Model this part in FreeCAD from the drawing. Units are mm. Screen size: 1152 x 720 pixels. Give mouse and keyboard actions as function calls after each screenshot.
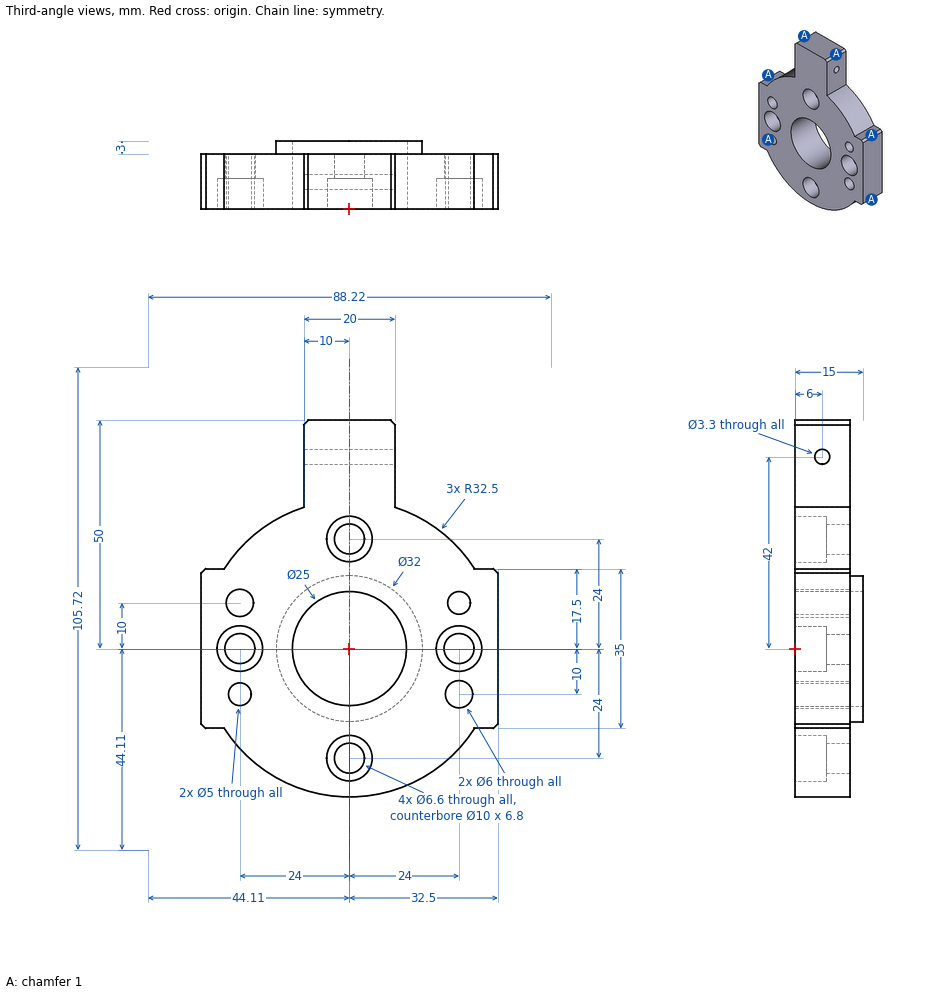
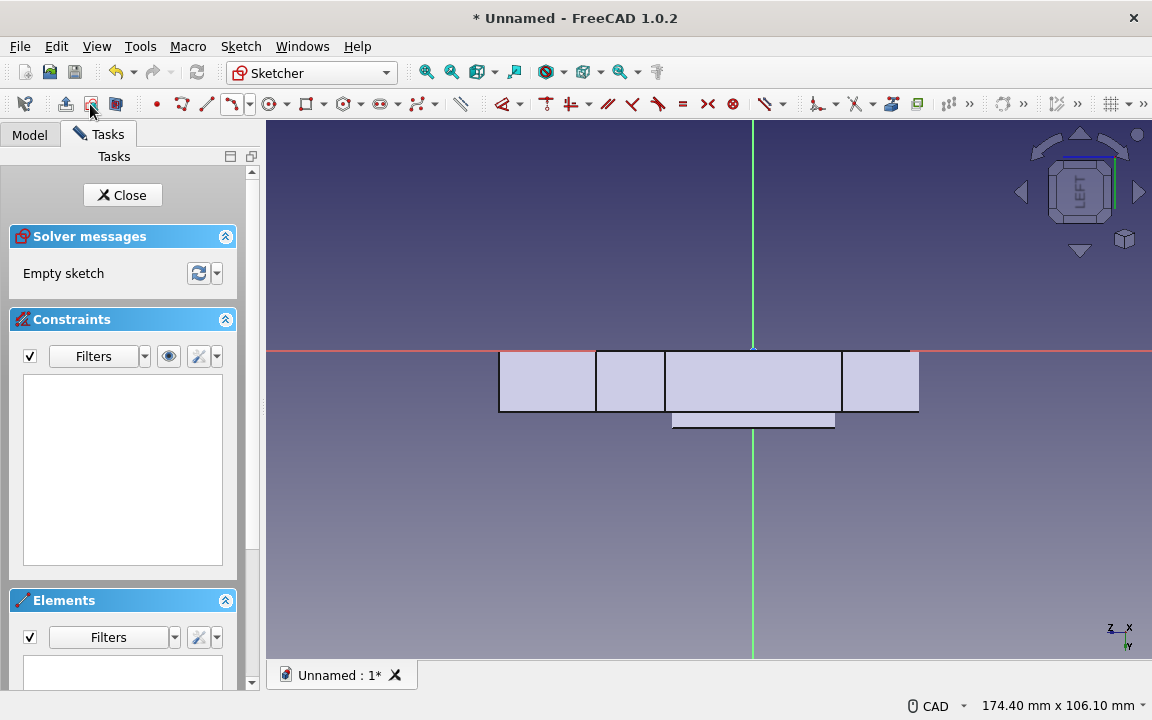
click(116, 104)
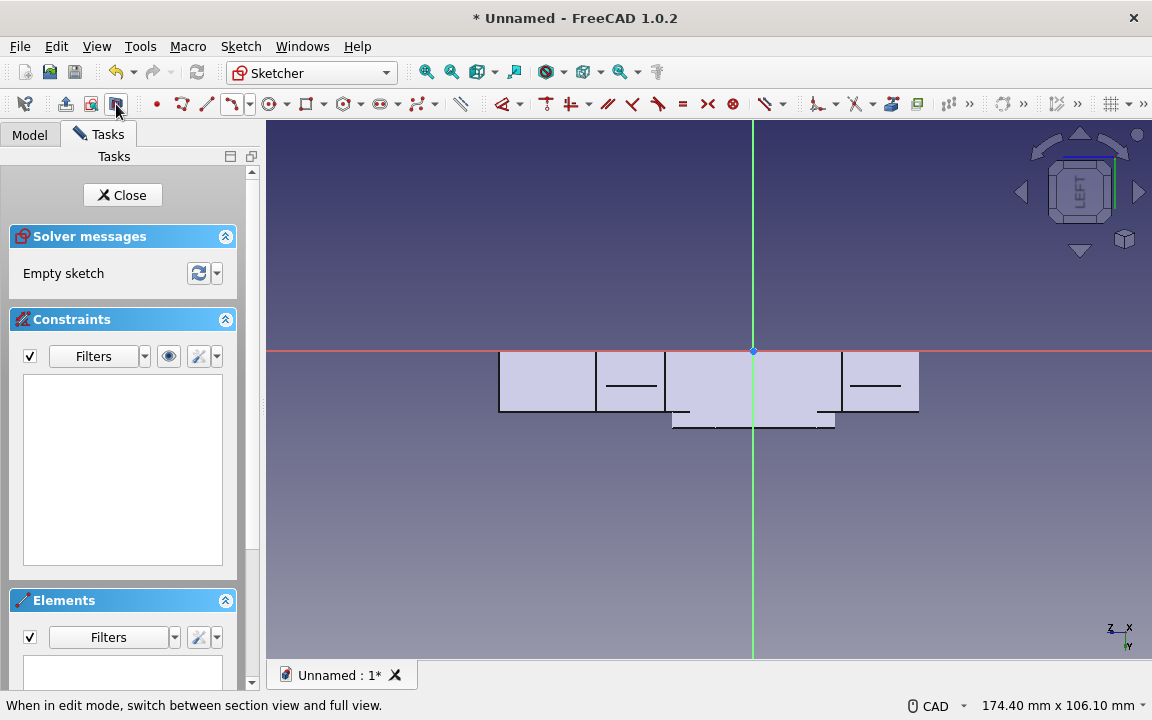
scroll(535, 381, up, 15)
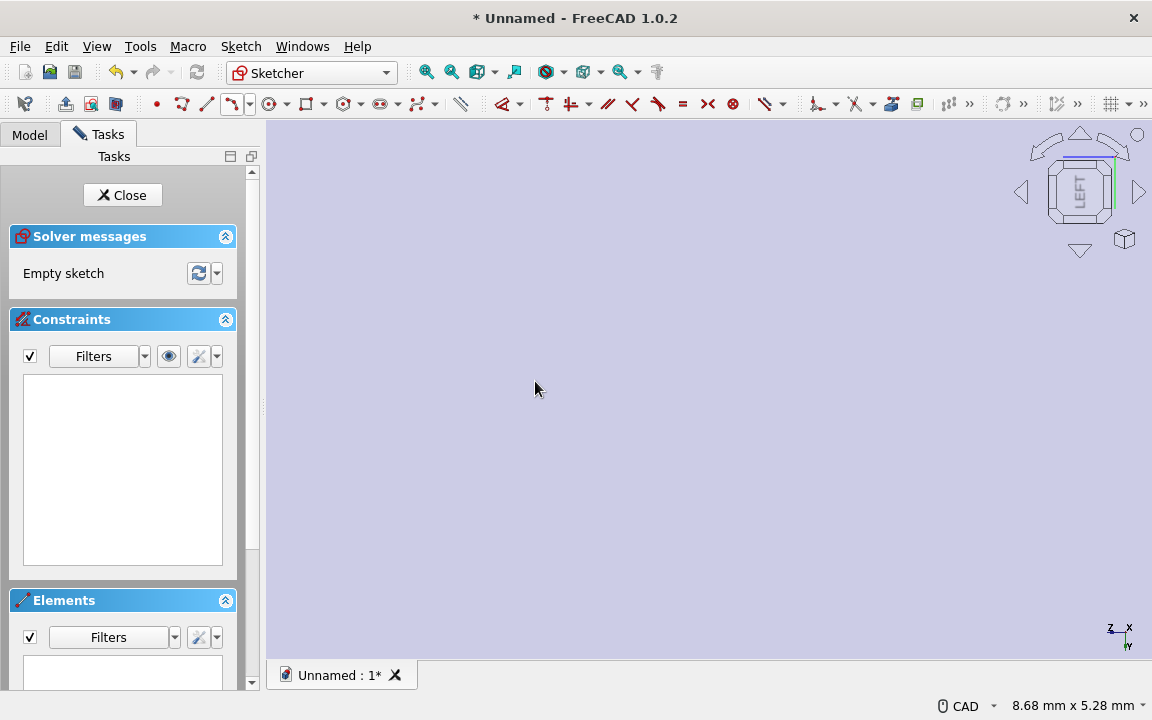
click(268, 104)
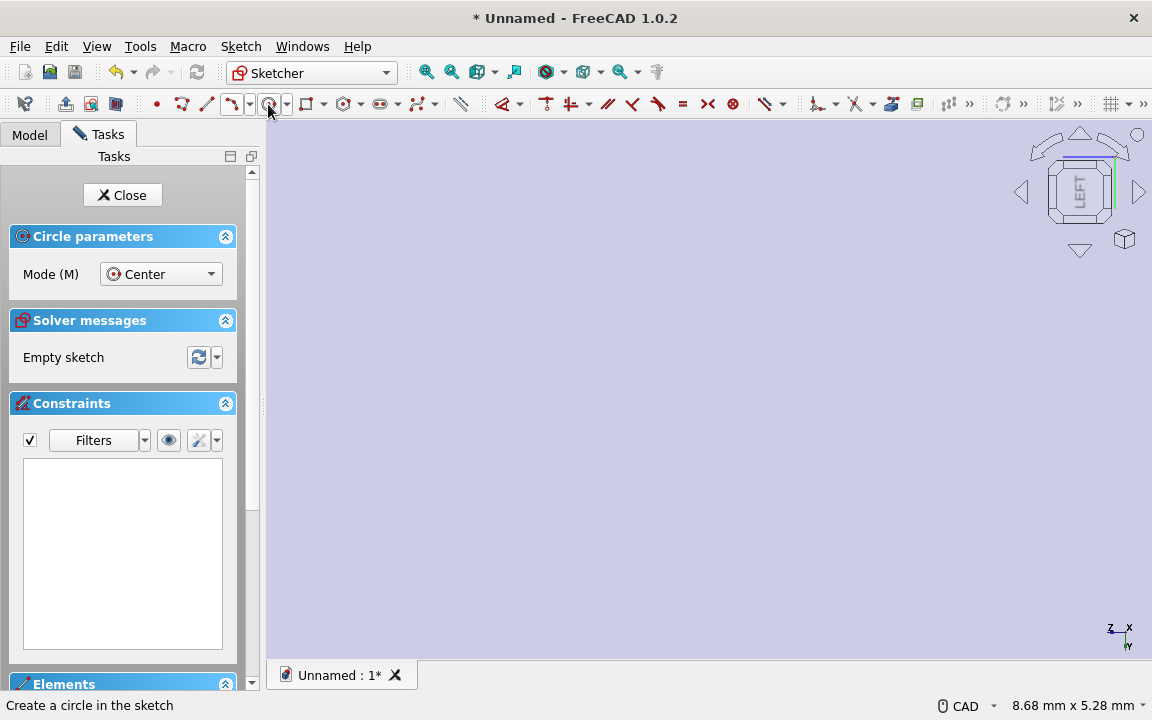
click(631, 389)
click(750, 270)
key(Escape)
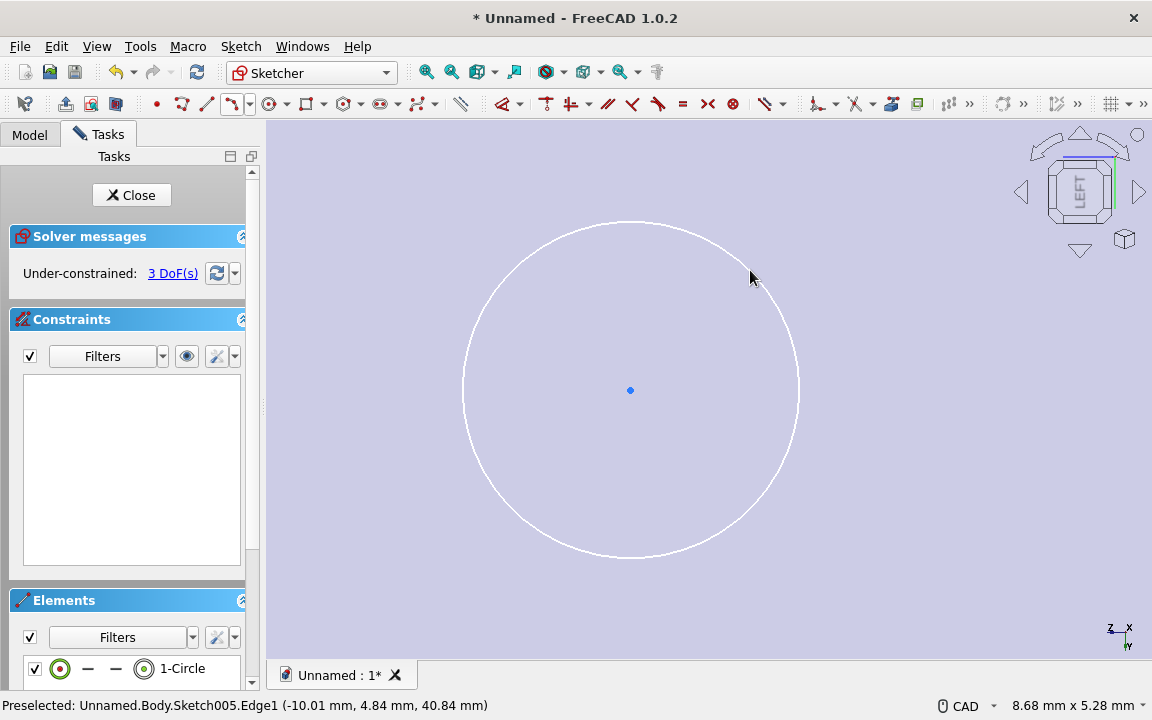
key(d)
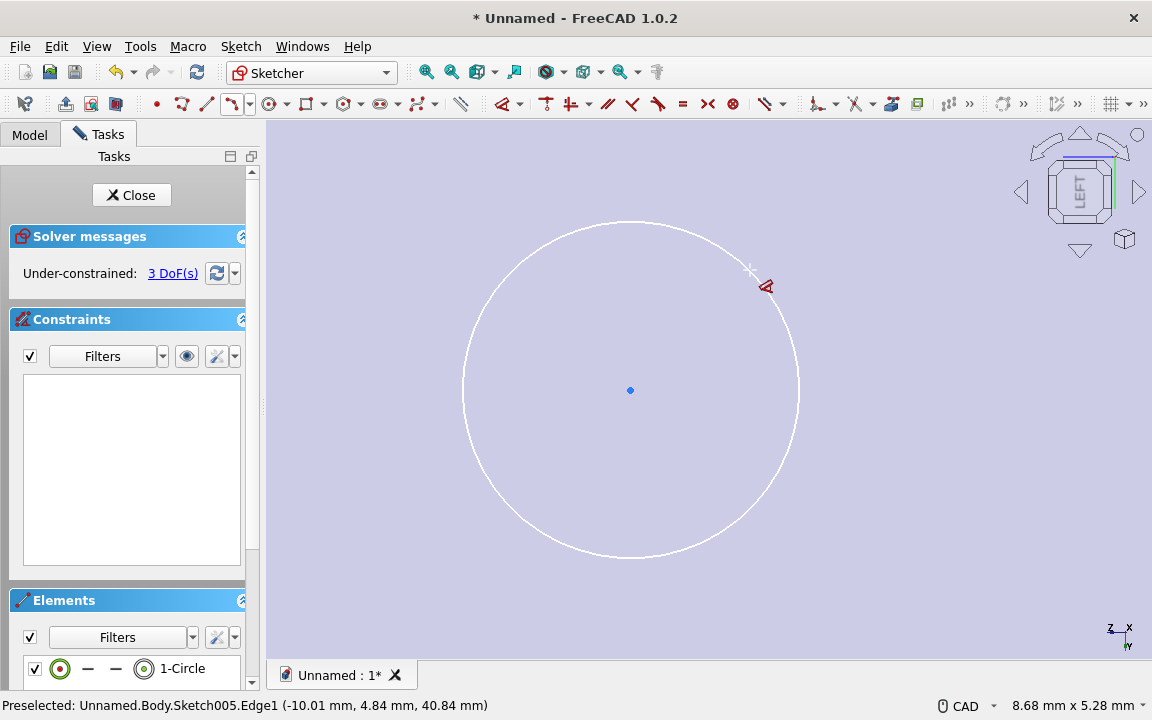
click(750, 271)
click(773, 248)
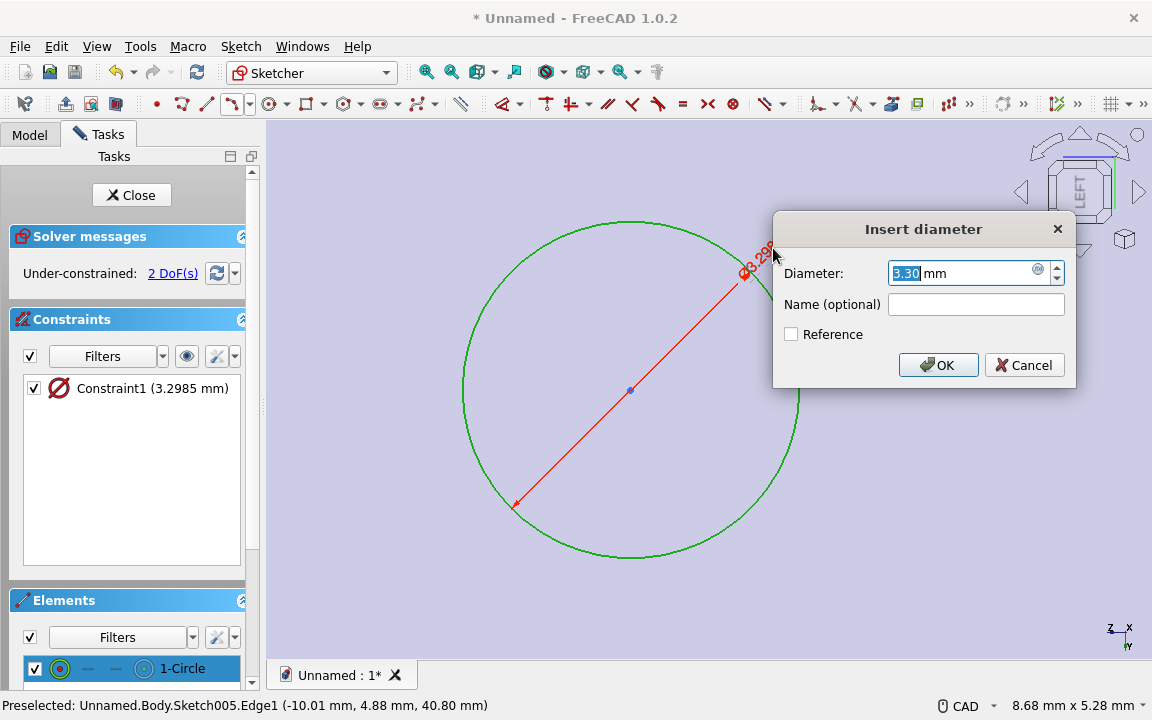
text(3.3)
key(Return)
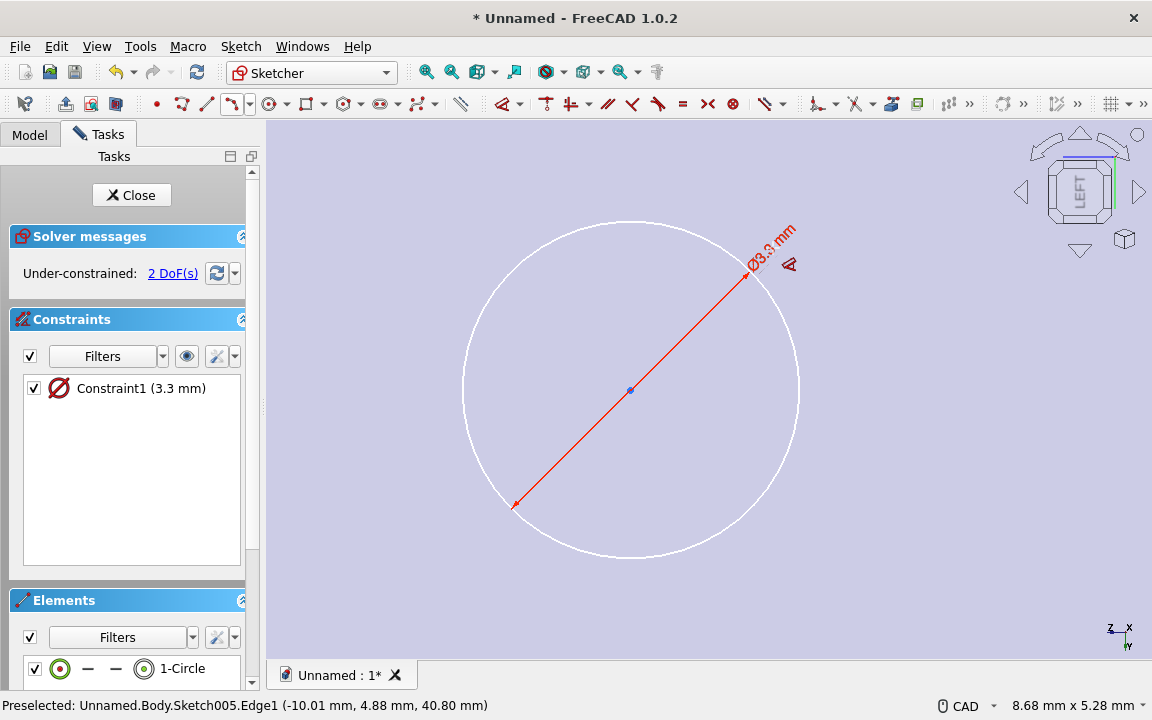
click(631, 390)
click(597, 269)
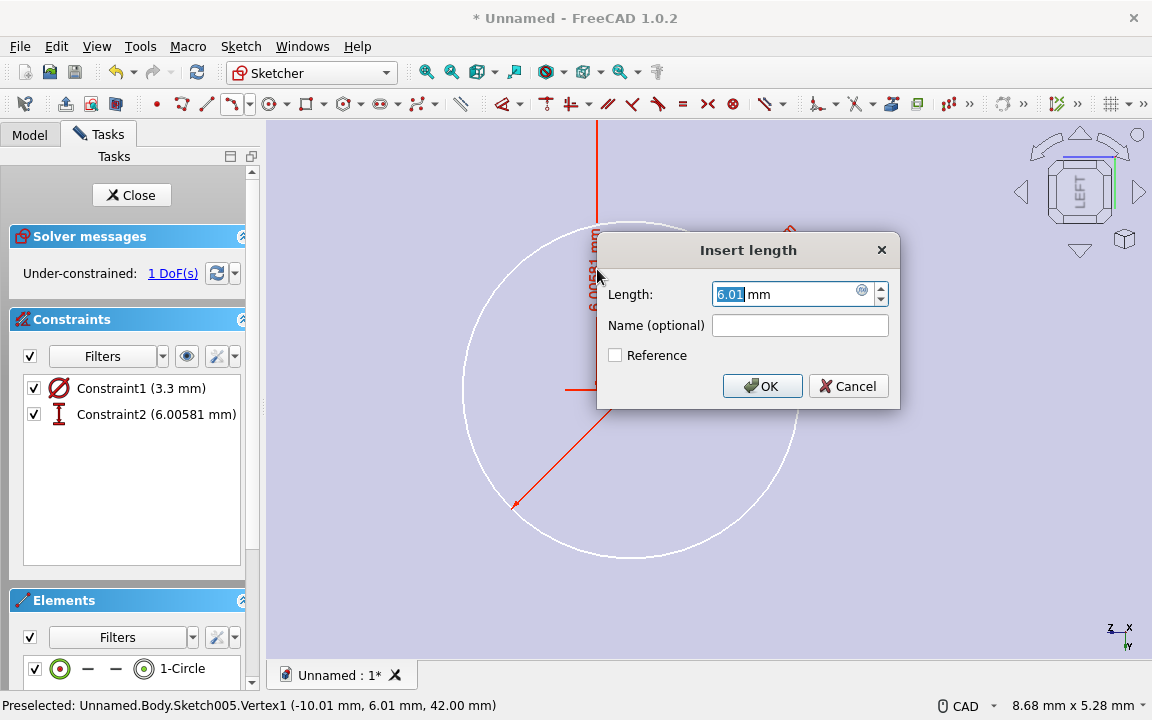
text(6)
key(Return)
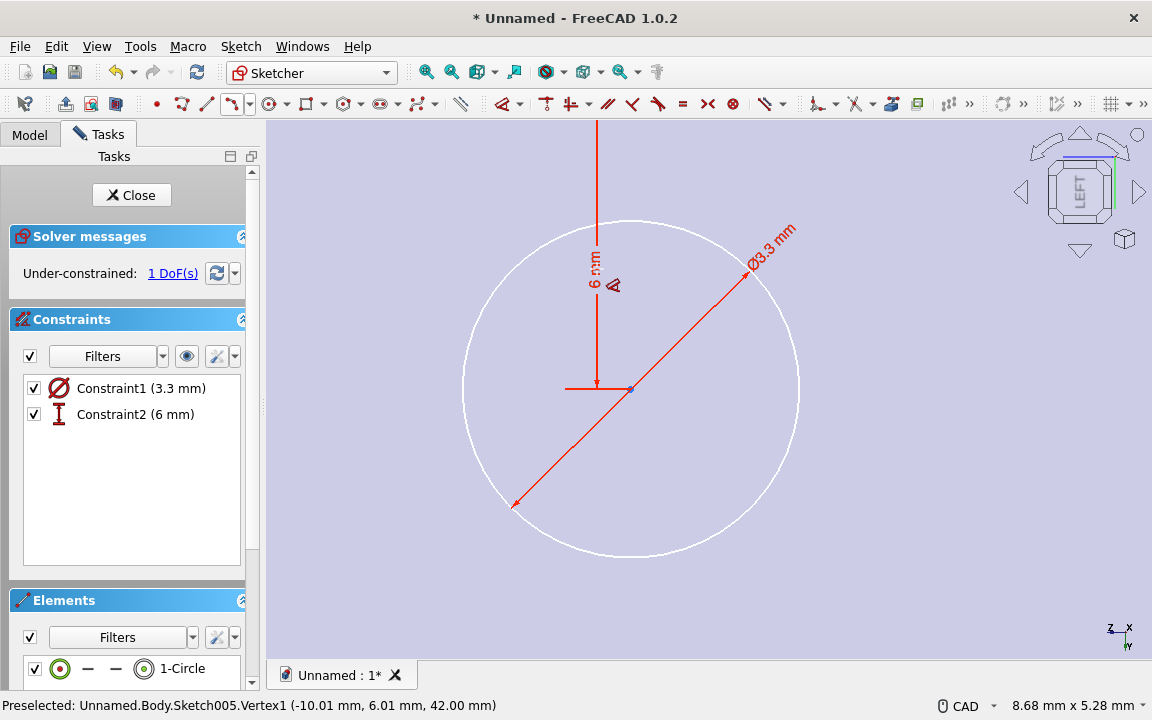
click(631, 389)
click(727, 423)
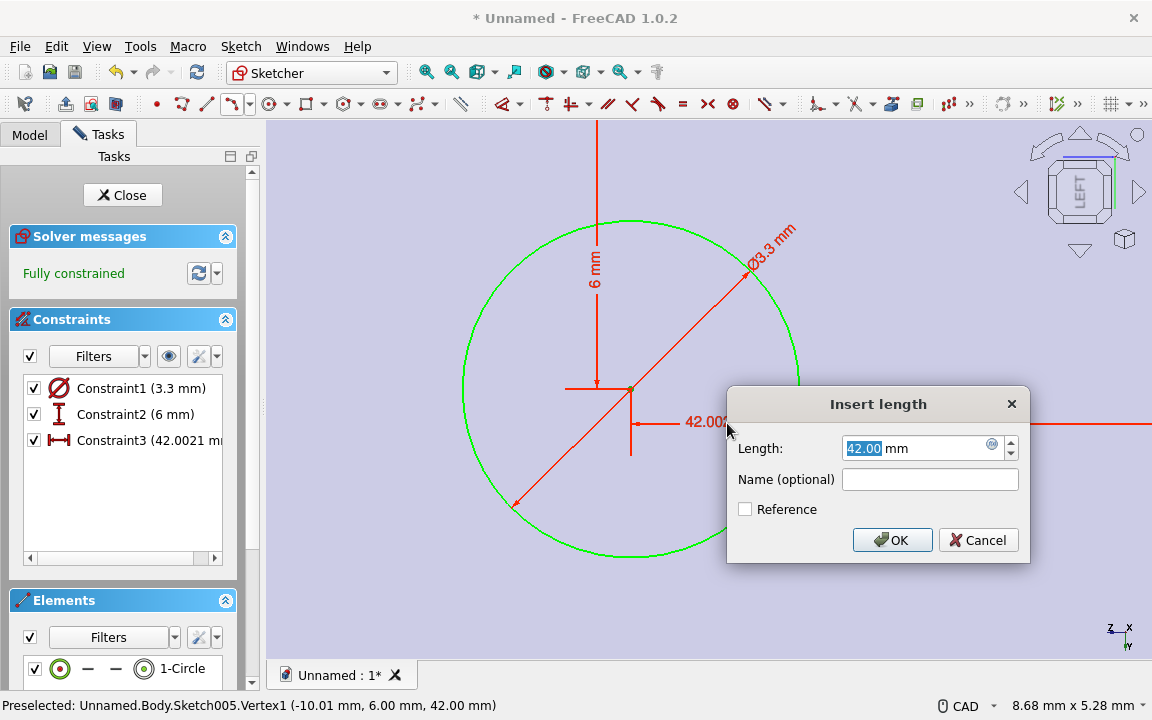
text(42)
key(Return)
key(Escape)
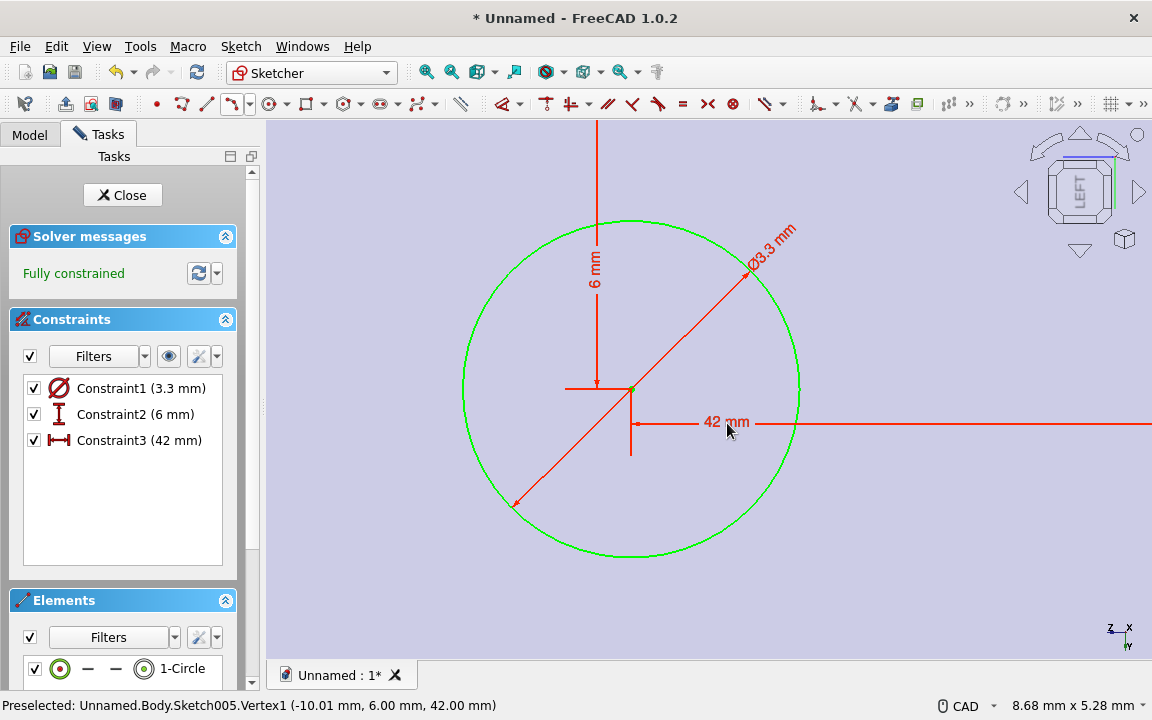
click(123, 195)